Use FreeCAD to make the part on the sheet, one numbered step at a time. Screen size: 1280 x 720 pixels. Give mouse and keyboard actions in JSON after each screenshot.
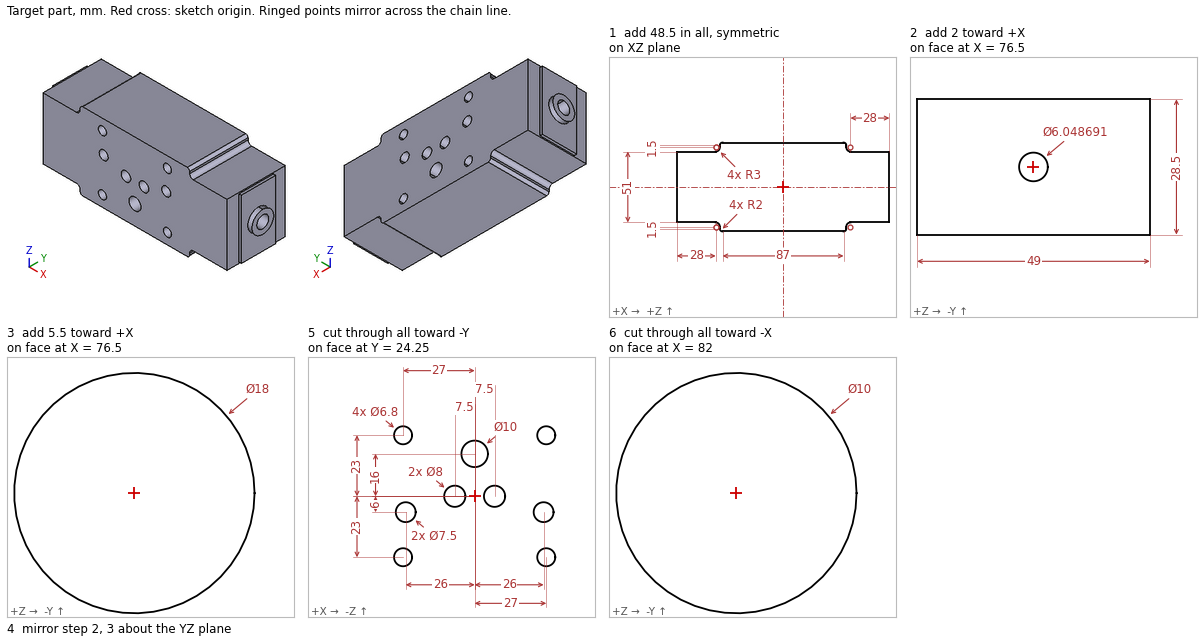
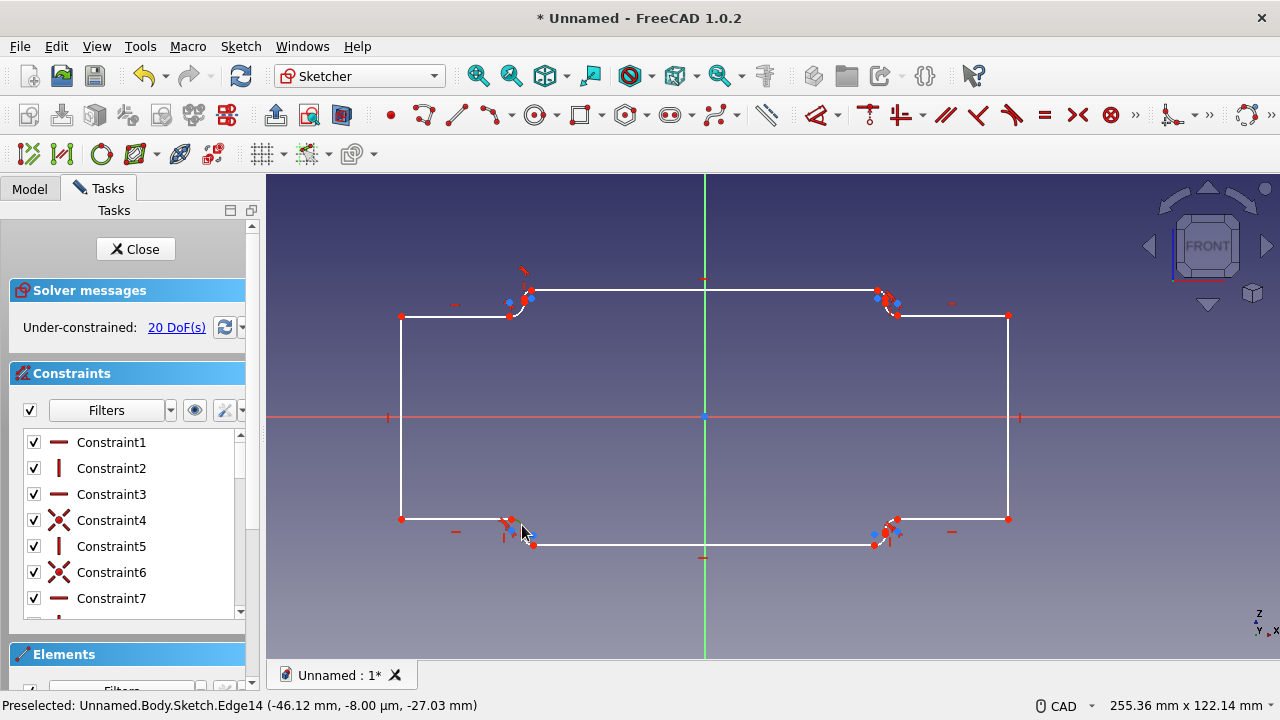
{"action": "scroll", "coordinate": [516, 315], "scroll_direction": "up", "scroll_amount": 4}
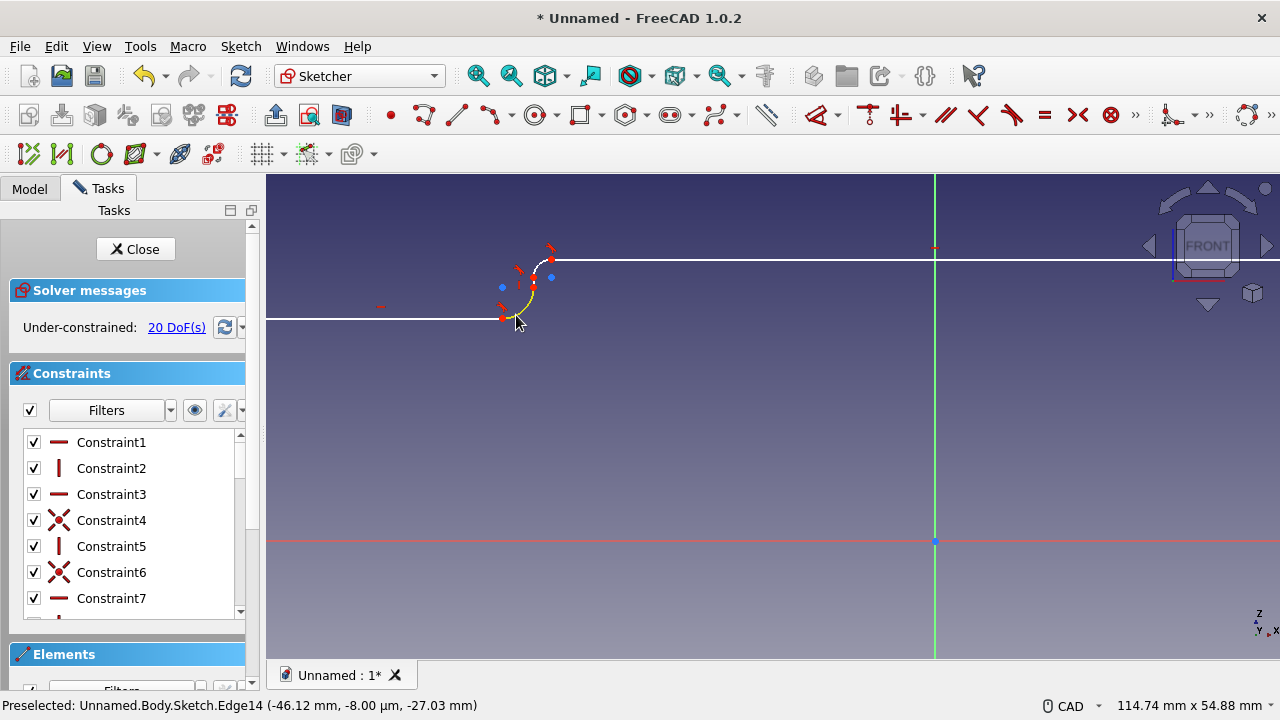
{"action": "left_click", "coordinate": [516, 315]}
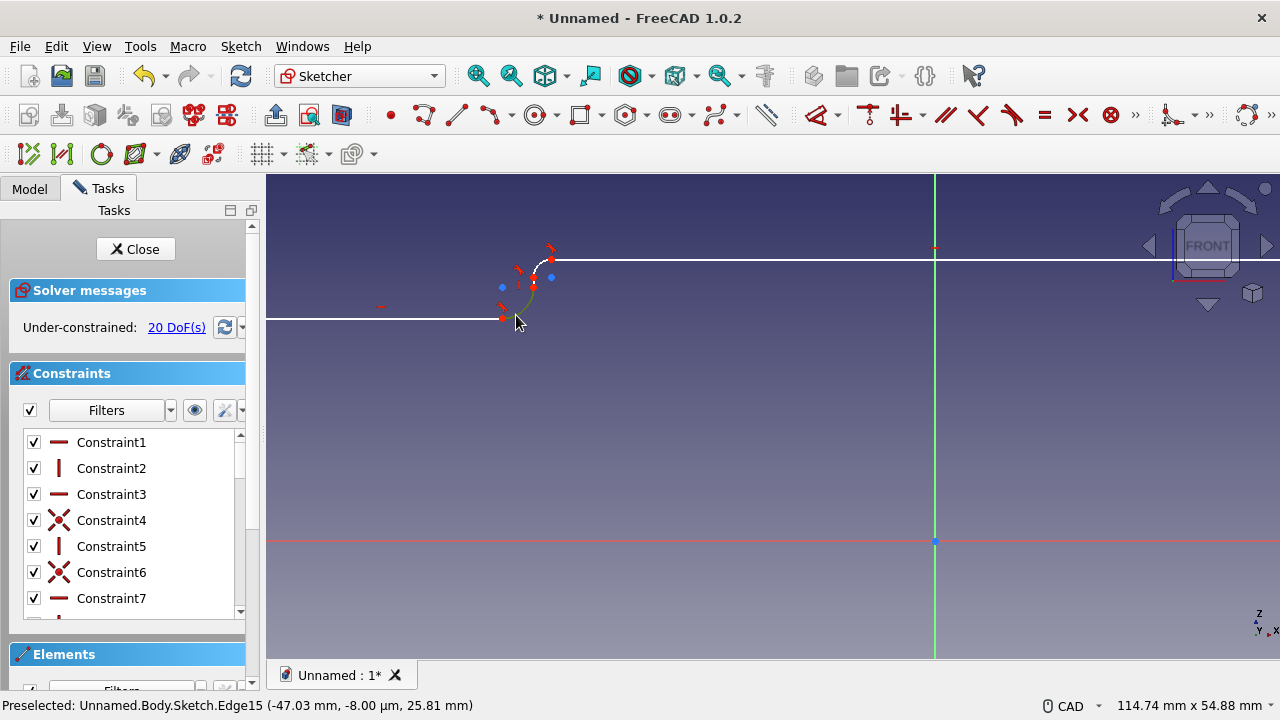
{"action": "scroll", "coordinate": [516, 315], "scroll_direction": "down", "scroll_amount": 4}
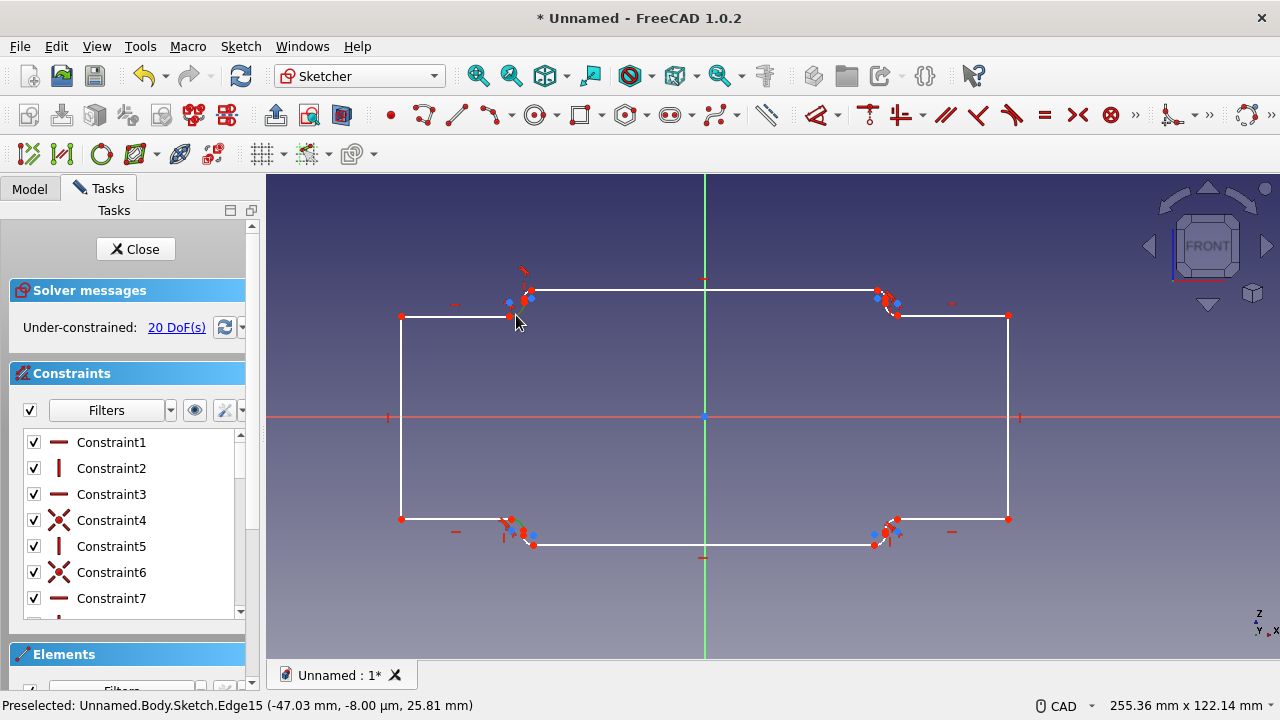
{"action": "scroll", "coordinate": [887, 309], "scroll_direction": "up", "scroll_amount": 5}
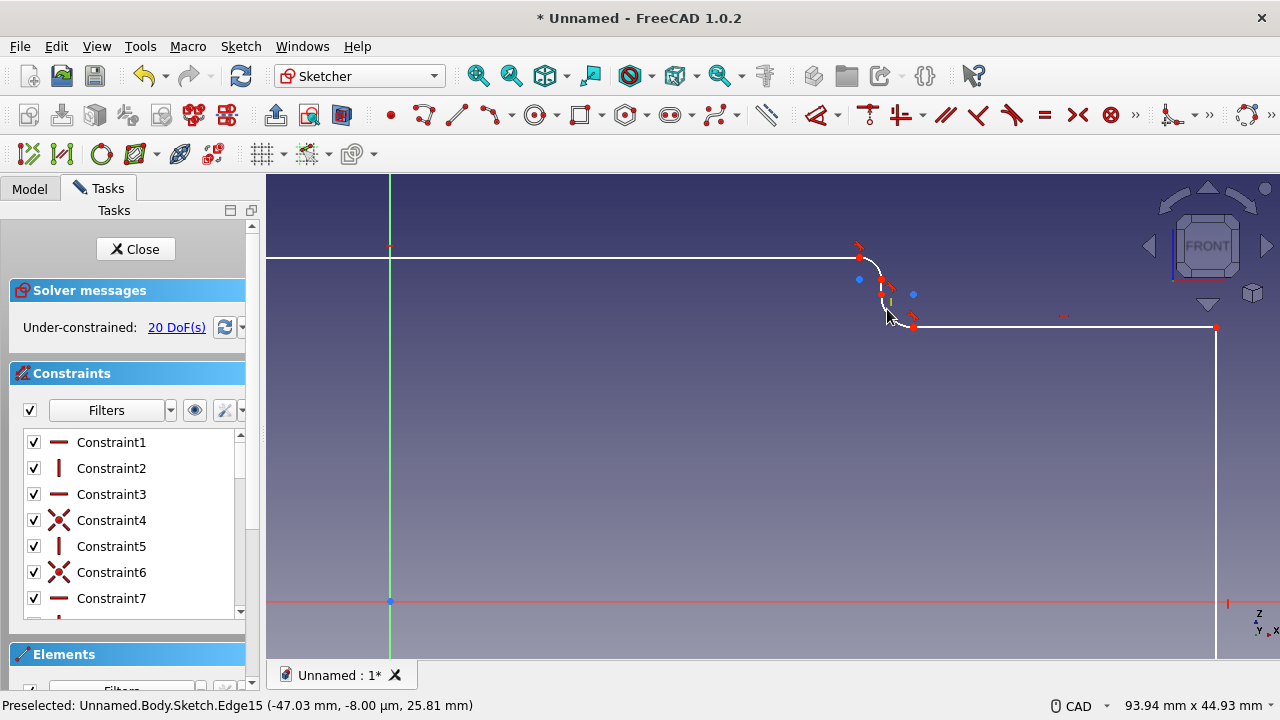
{"action": "left_click", "coordinate": [885, 310]}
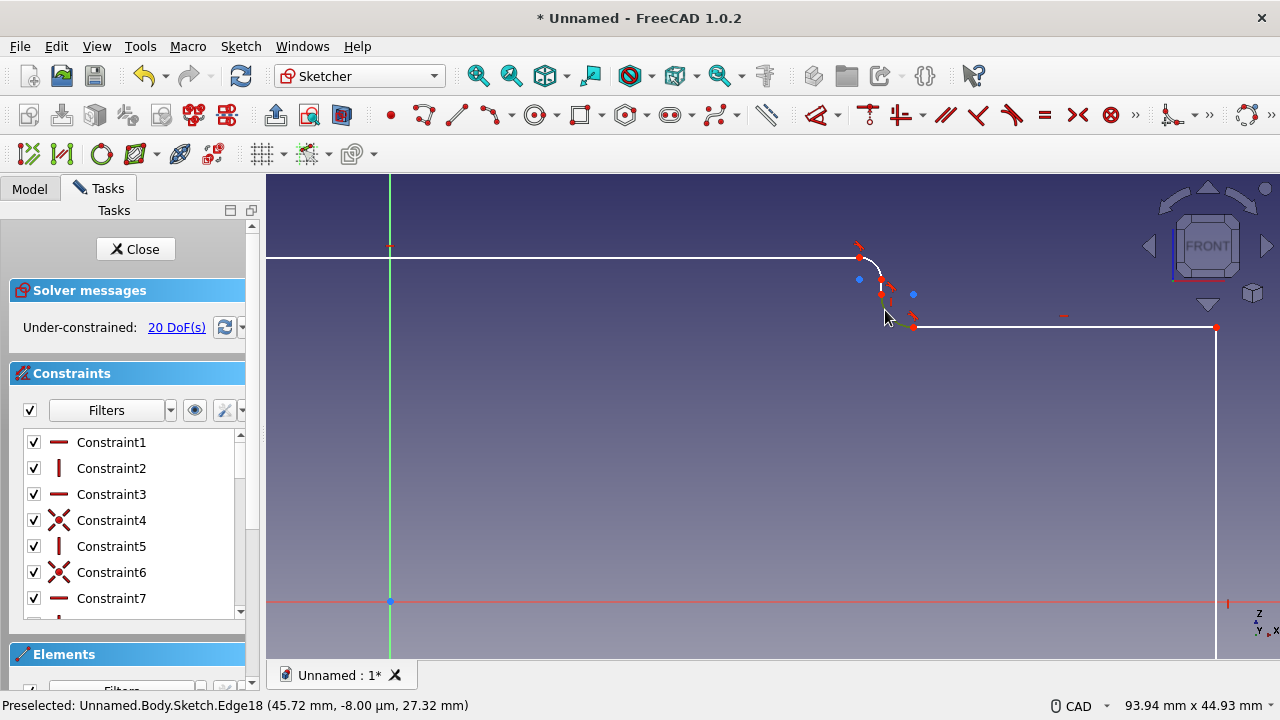
{"action": "scroll", "coordinate": [887, 309], "scroll_direction": "down", "scroll_amount": 5}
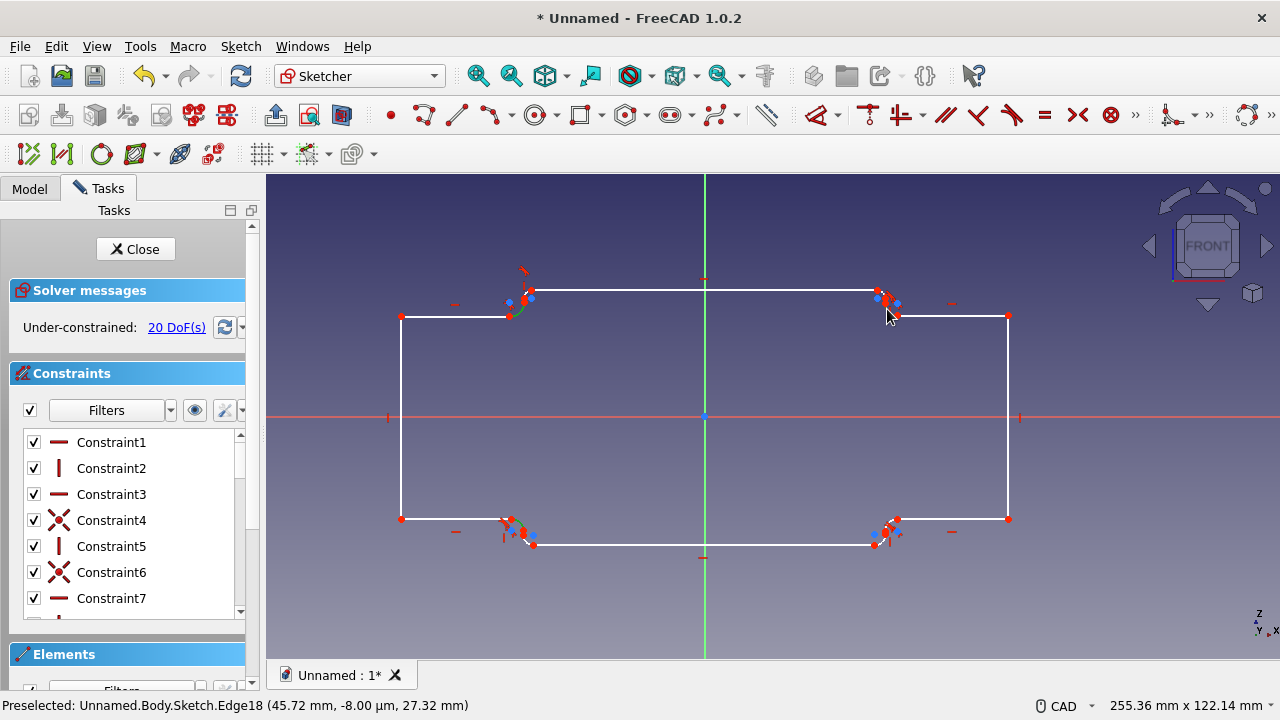
{"action": "scroll", "coordinate": [892, 520], "scroll_direction": "up", "scroll_amount": 5}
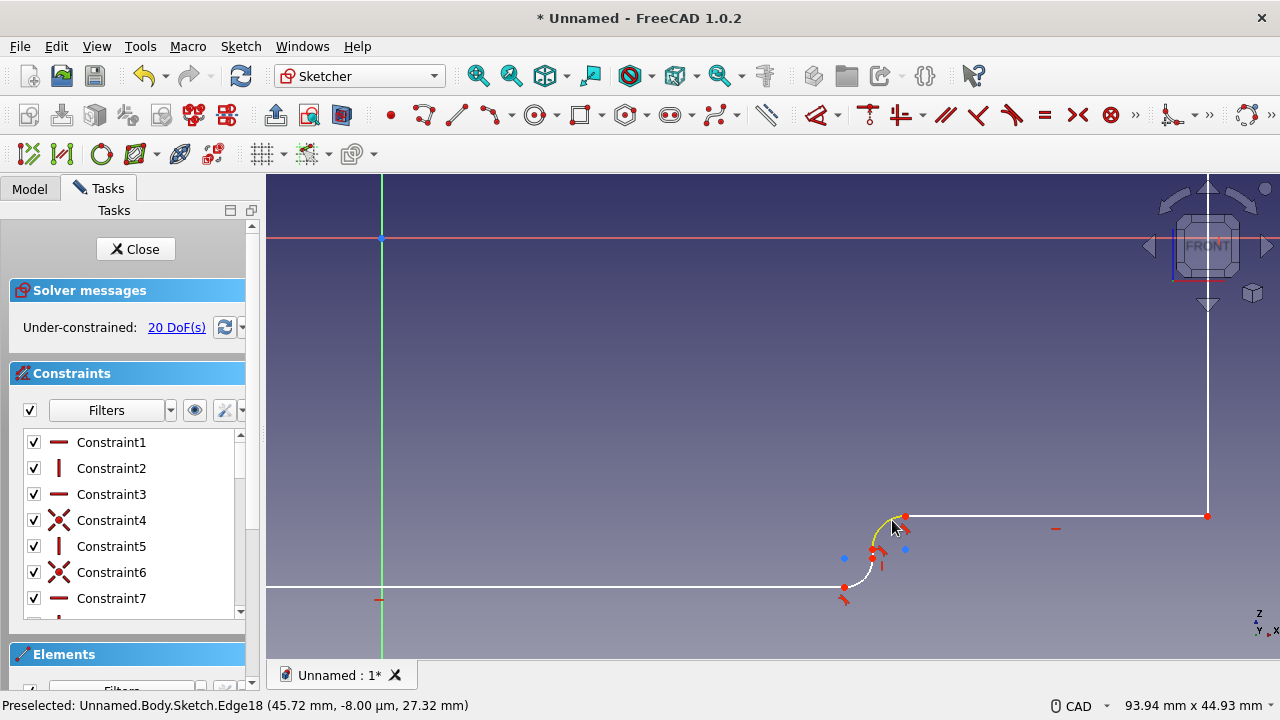
{"action": "left_click", "coordinate": [891, 520]}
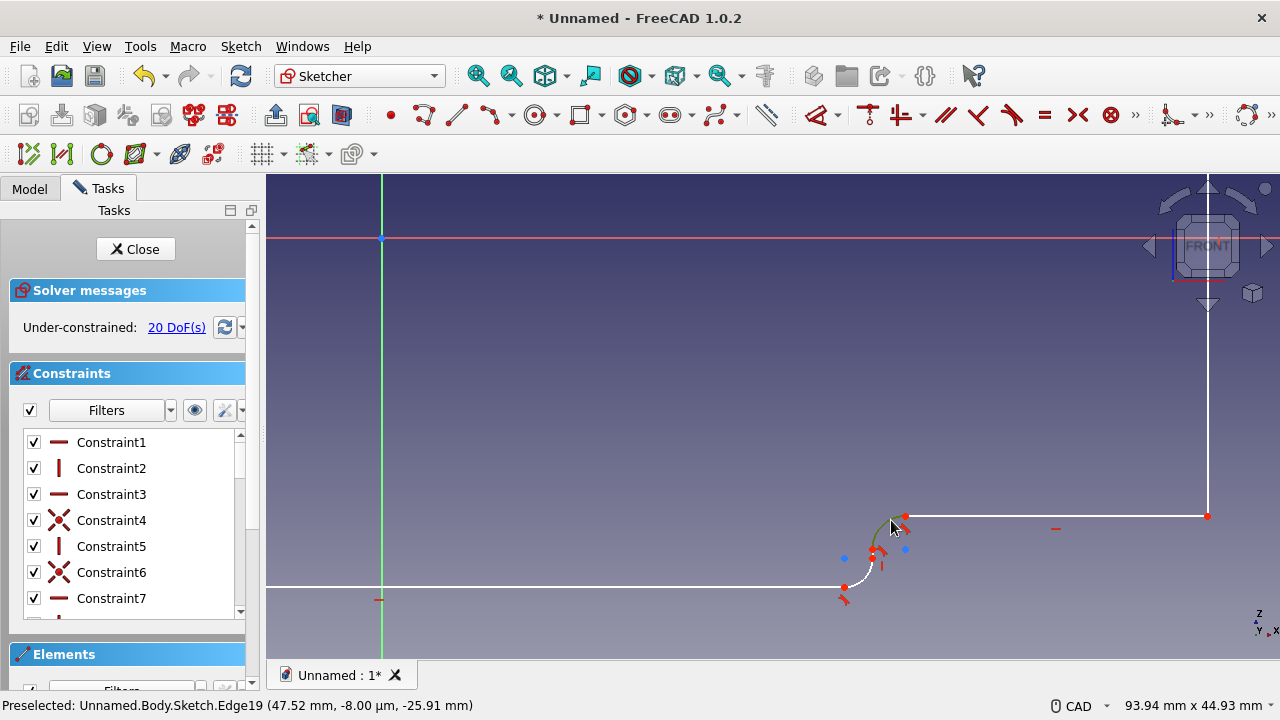
{"action": "left_click", "coordinate": [1045, 116]}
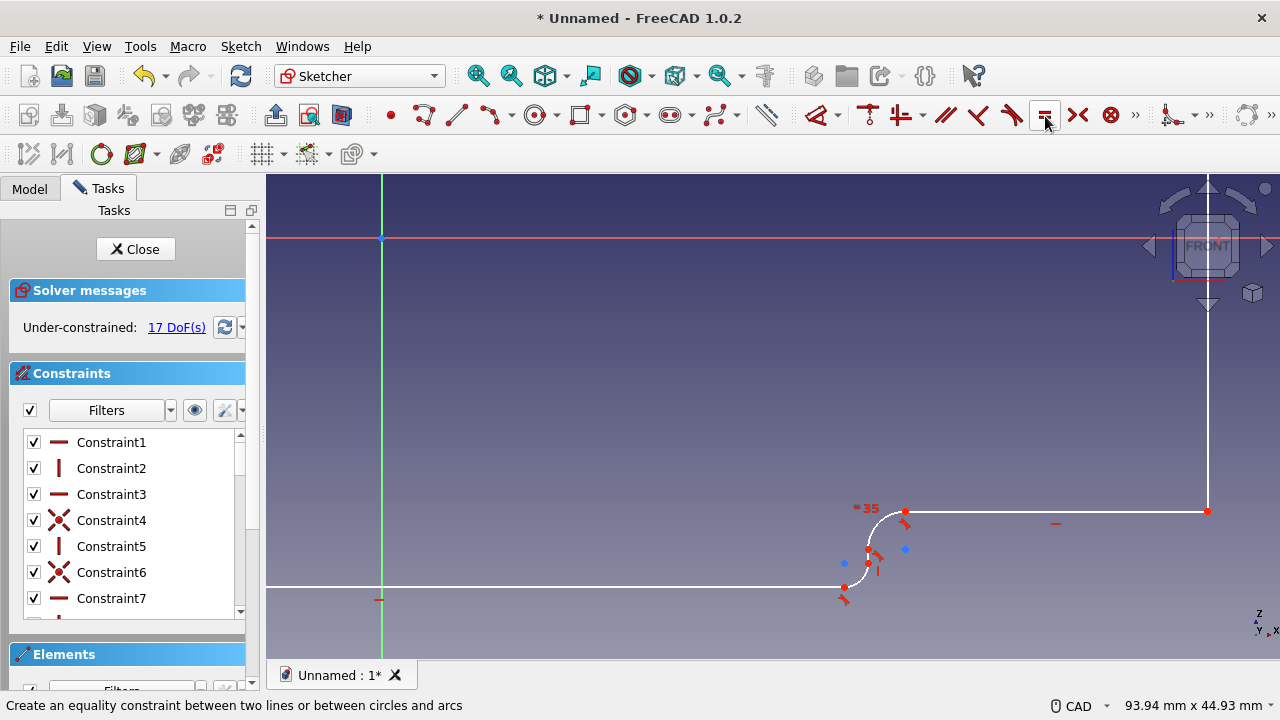
{"action": "scroll", "coordinate": [892, 520], "scroll_direction": "down", "scroll_amount": 5}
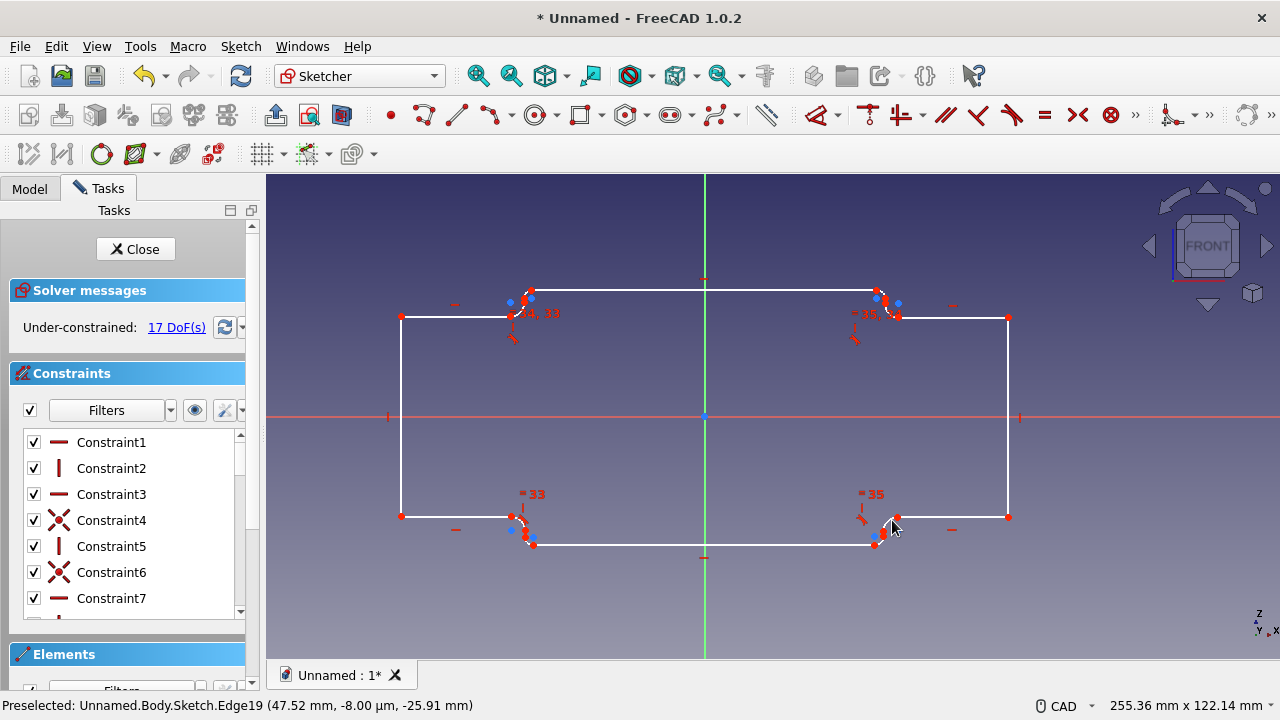
{"action": "scroll", "coordinate": [526, 541], "scroll_direction": "up", "scroll_amount": 7}